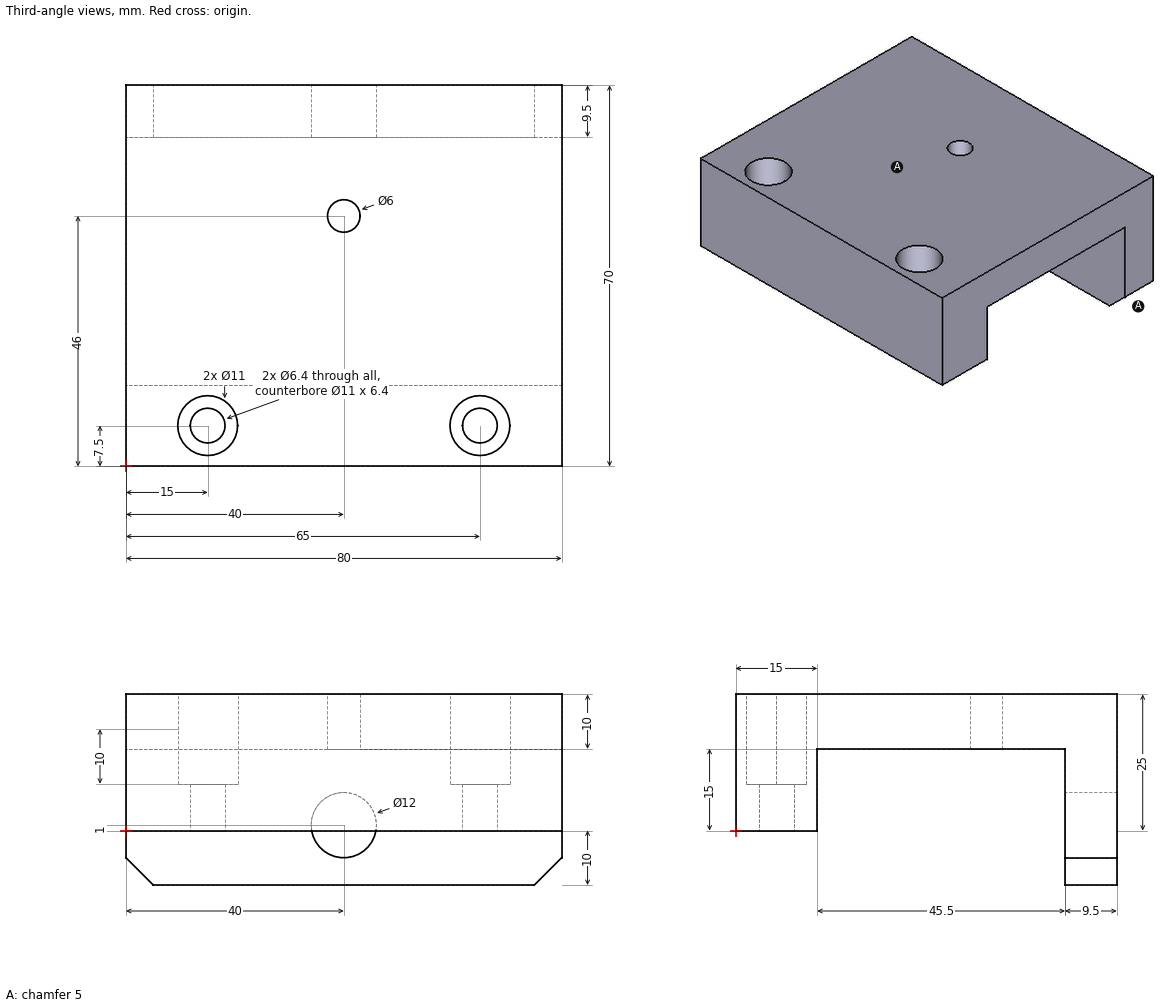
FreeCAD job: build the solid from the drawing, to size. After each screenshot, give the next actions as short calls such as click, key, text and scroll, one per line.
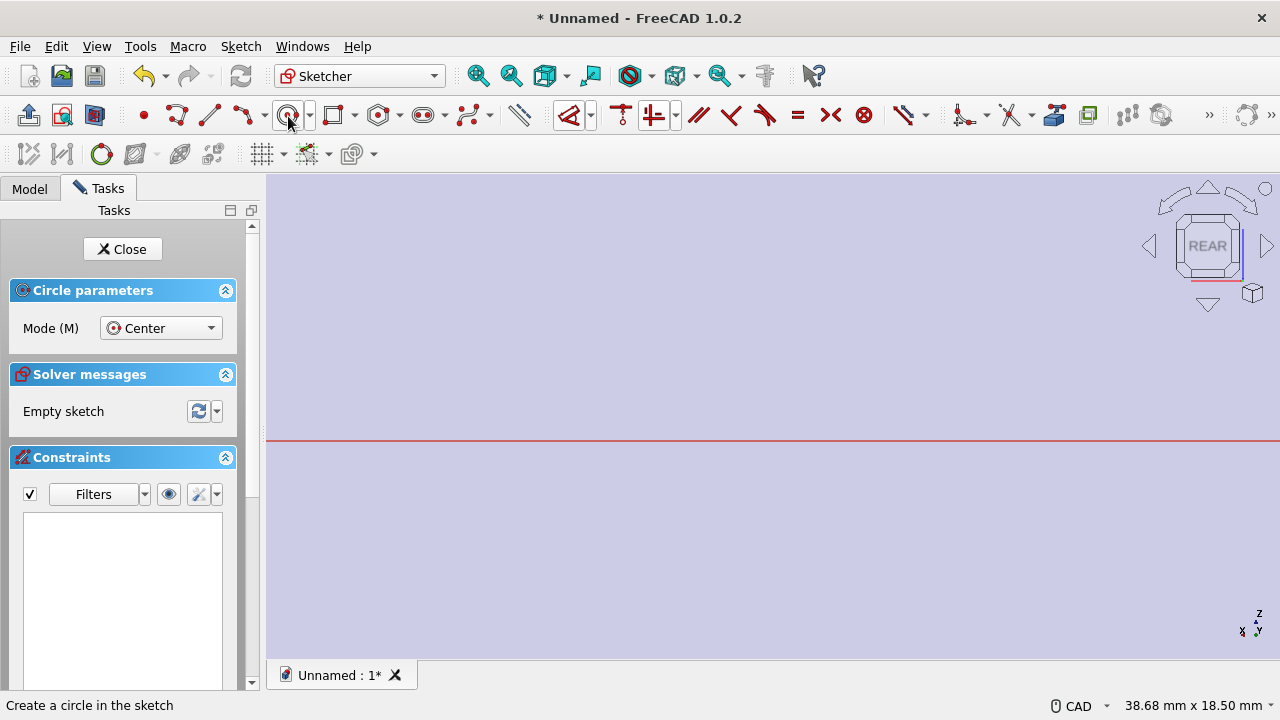
click(700, 415)
move(811, 304)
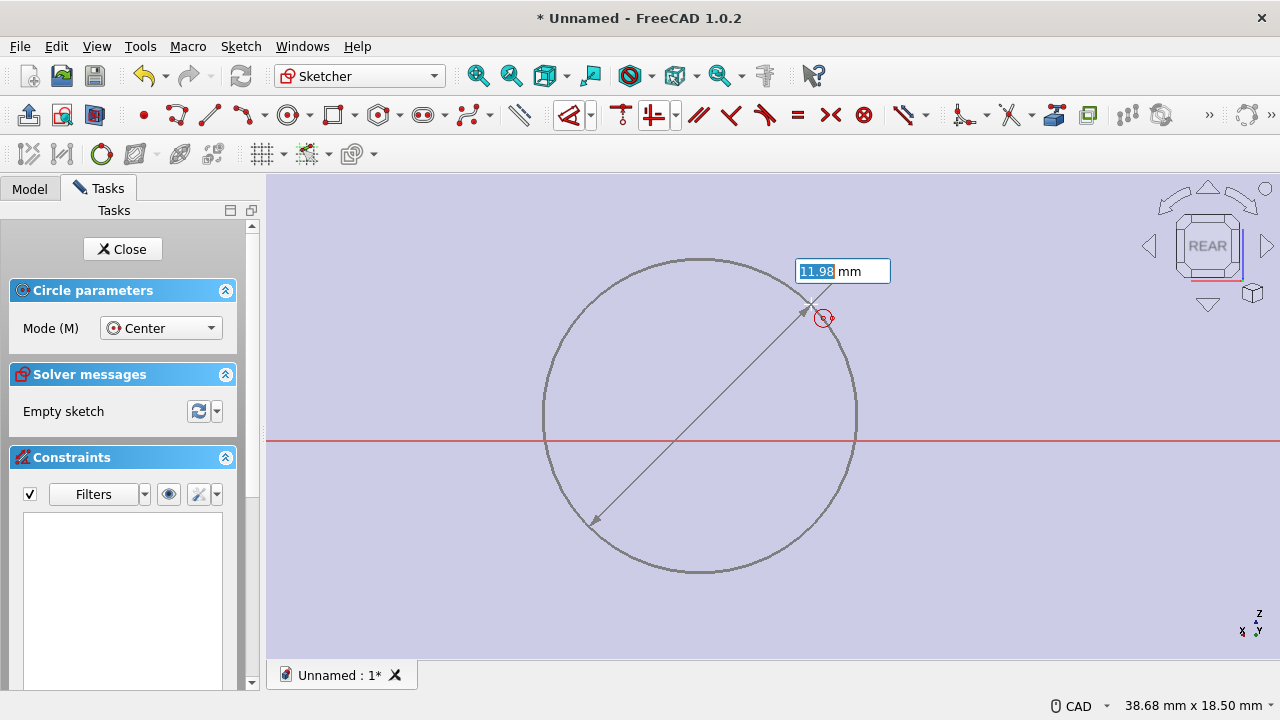
text(12)
key(Return)
key(Escape)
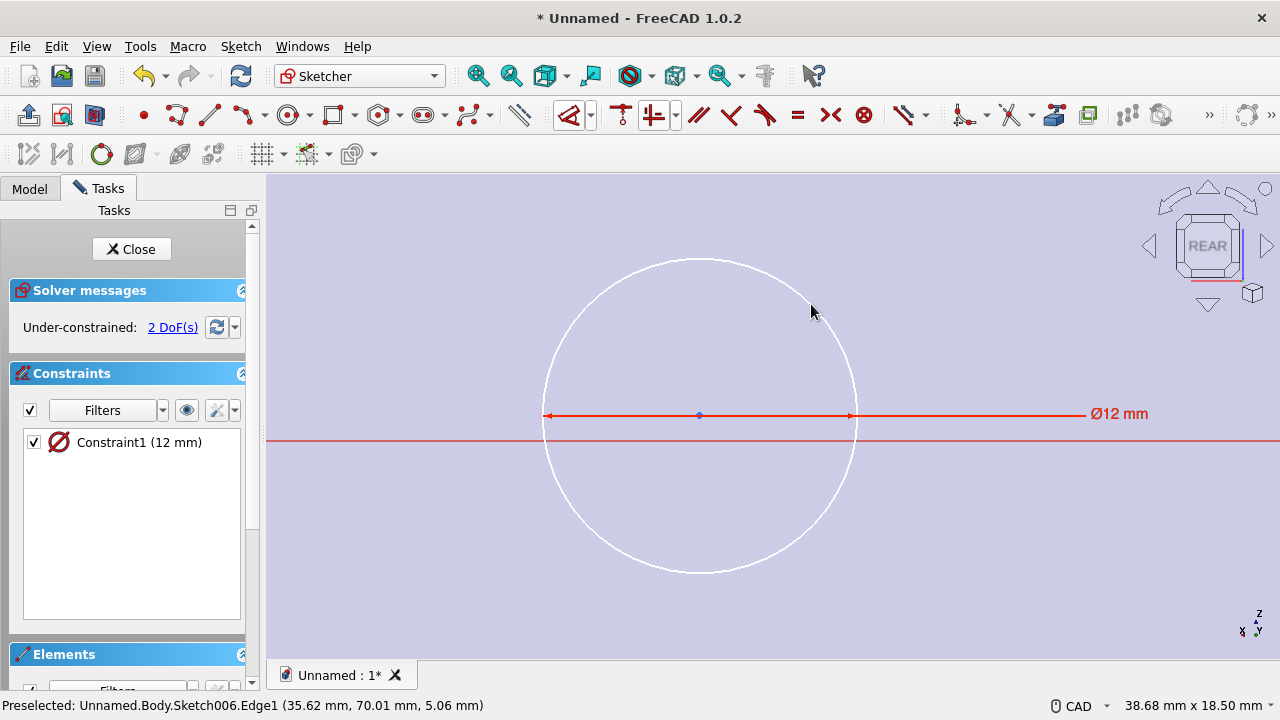
scroll(700, 416, up, 3)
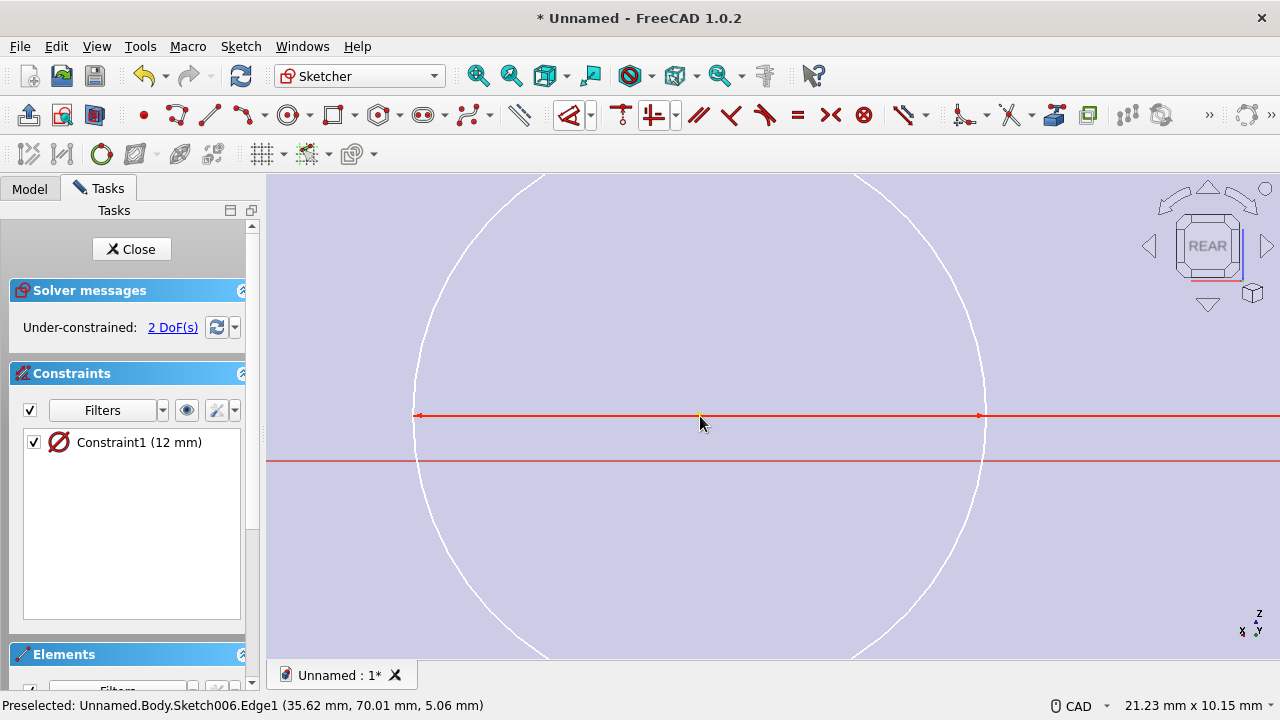
click(700, 416)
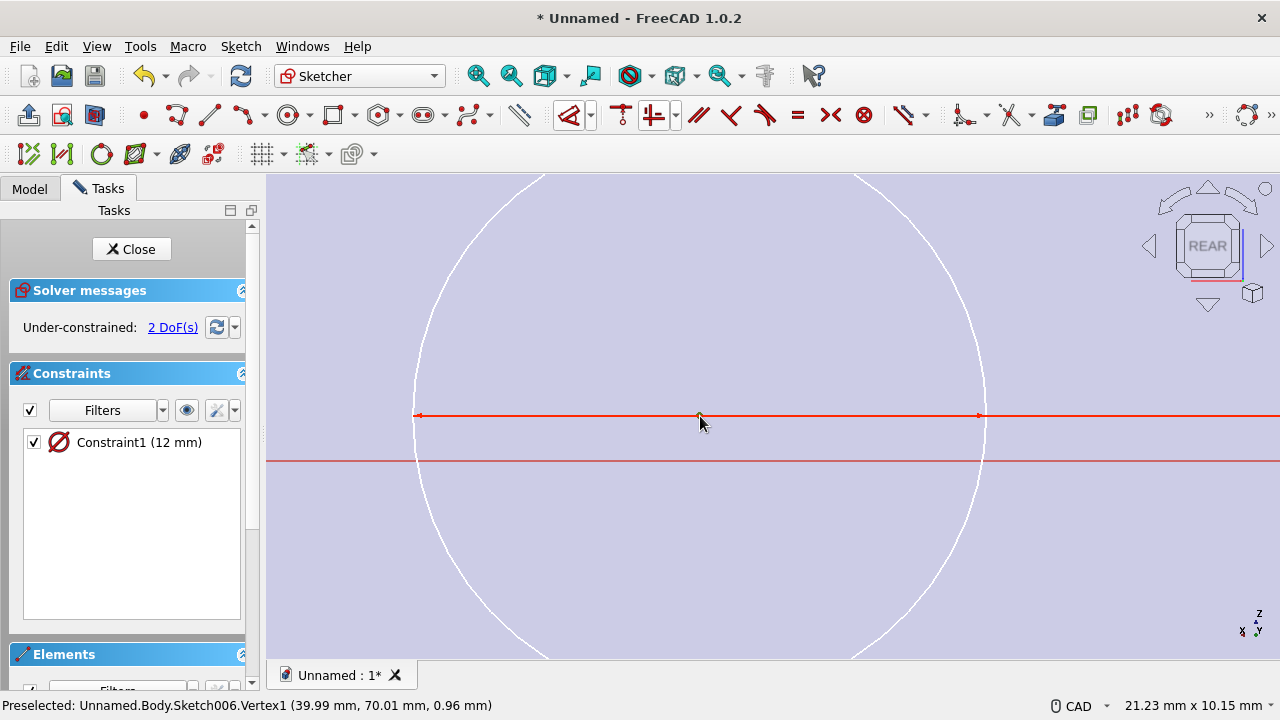
click(590, 116)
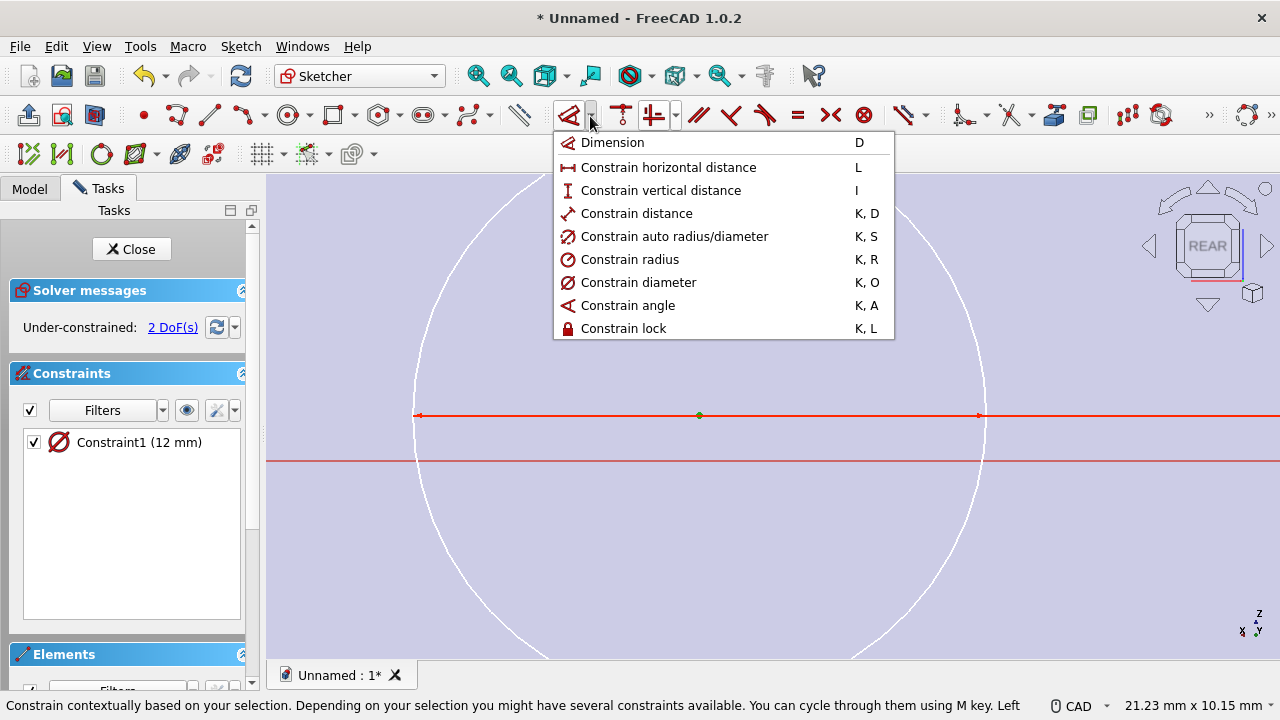
click(724, 190)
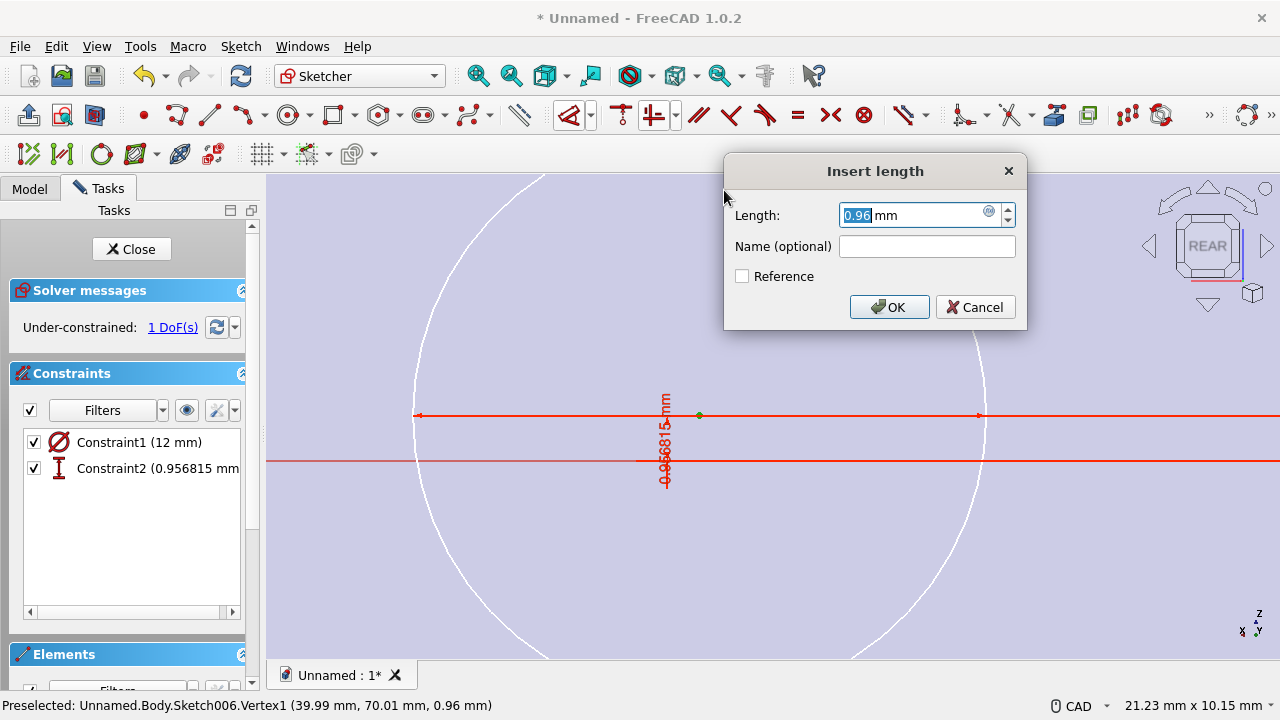
text(1)
key(Return)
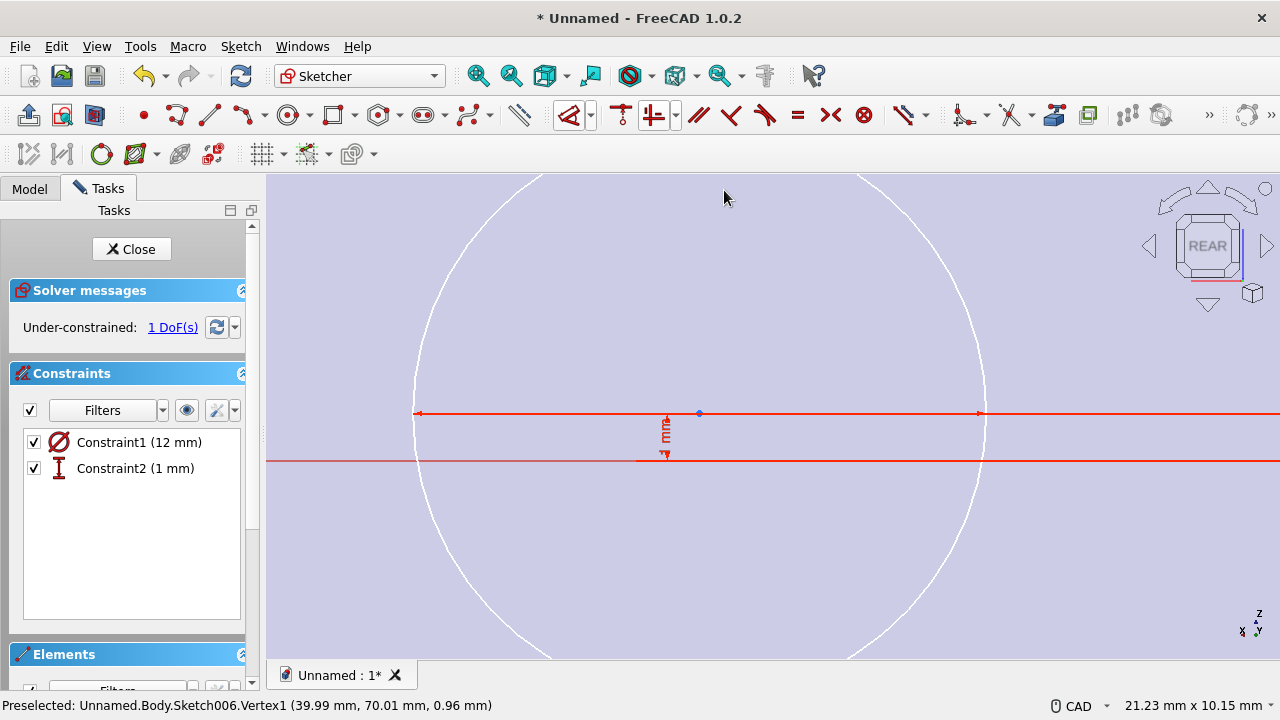
click(700, 414)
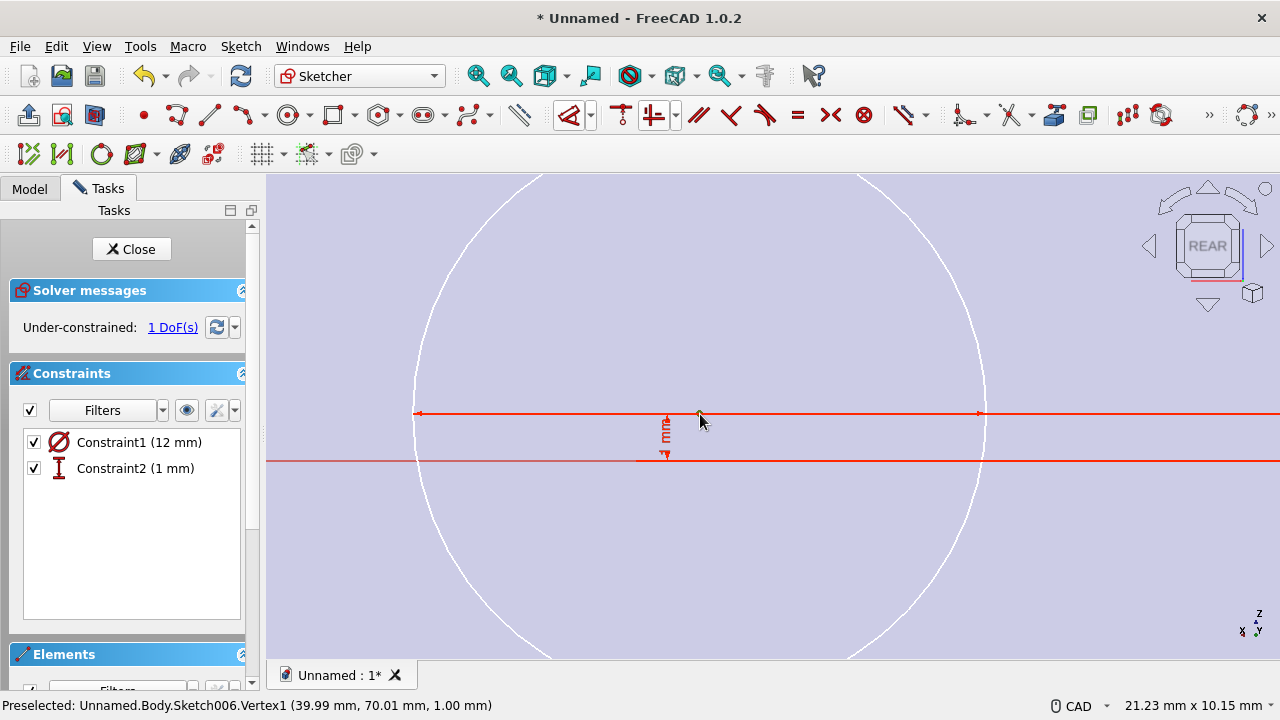
click(590, 116)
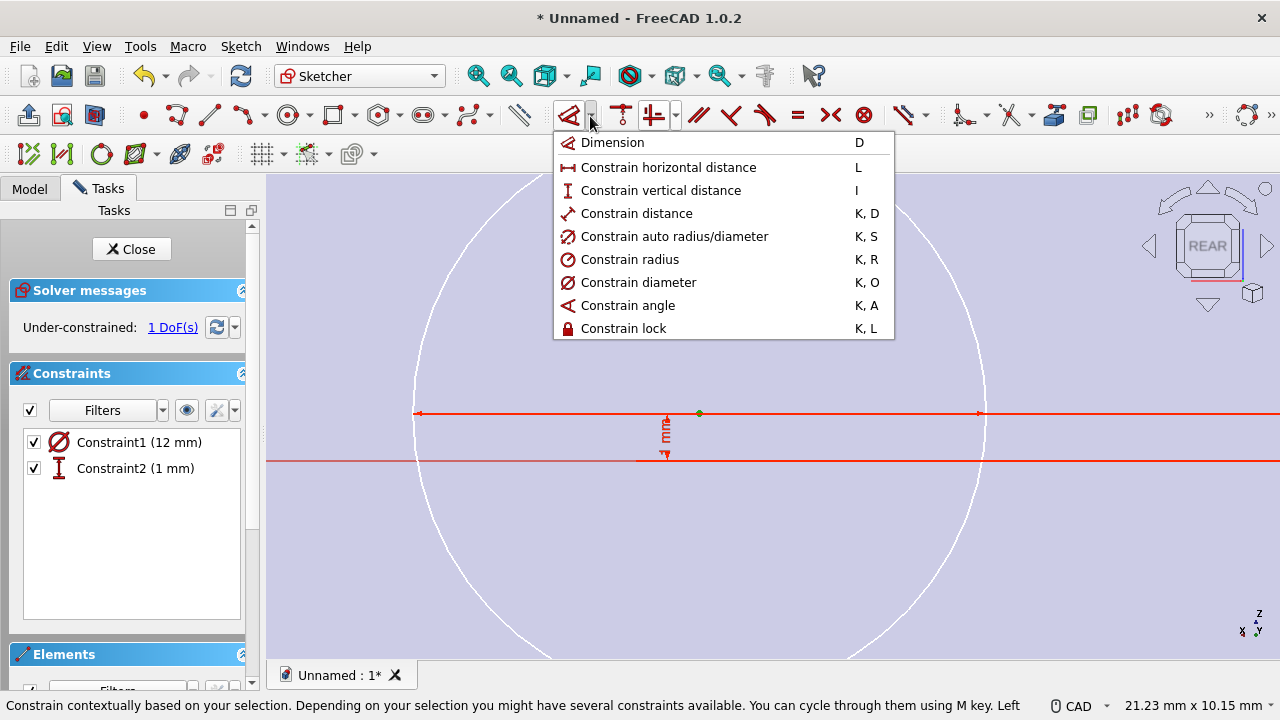
click(724, 168)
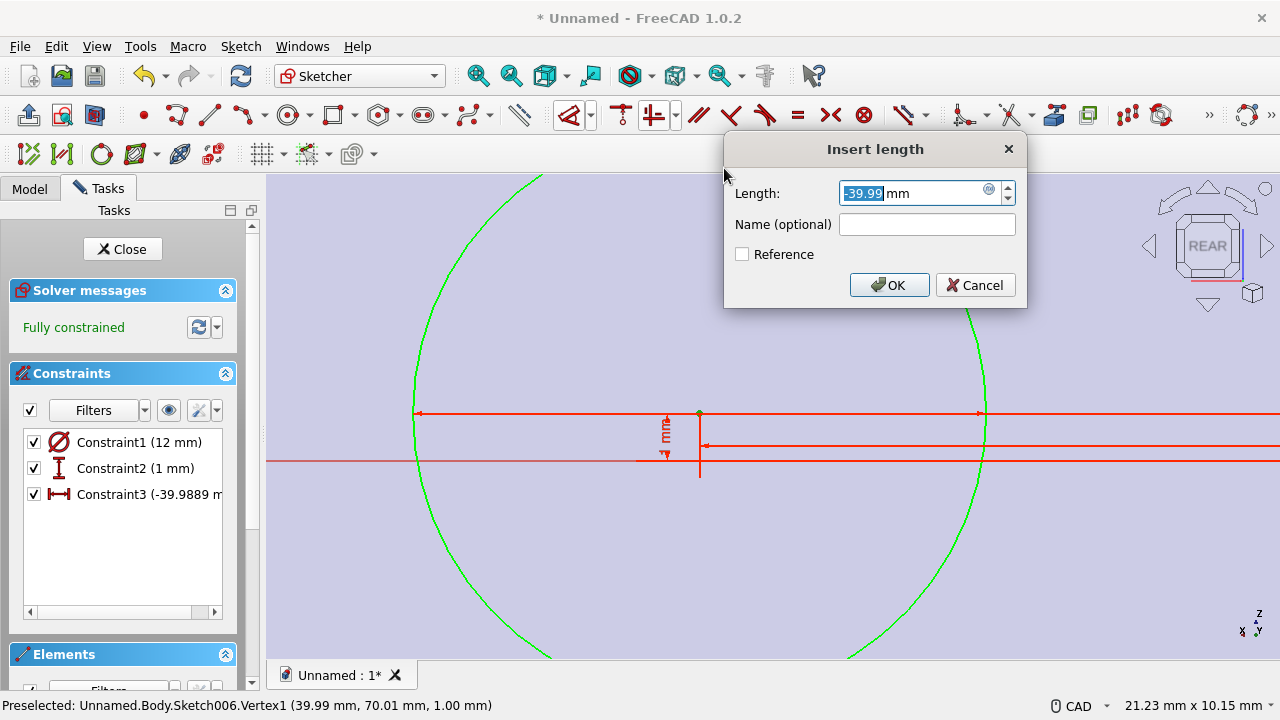
text(-40)
key(Return)